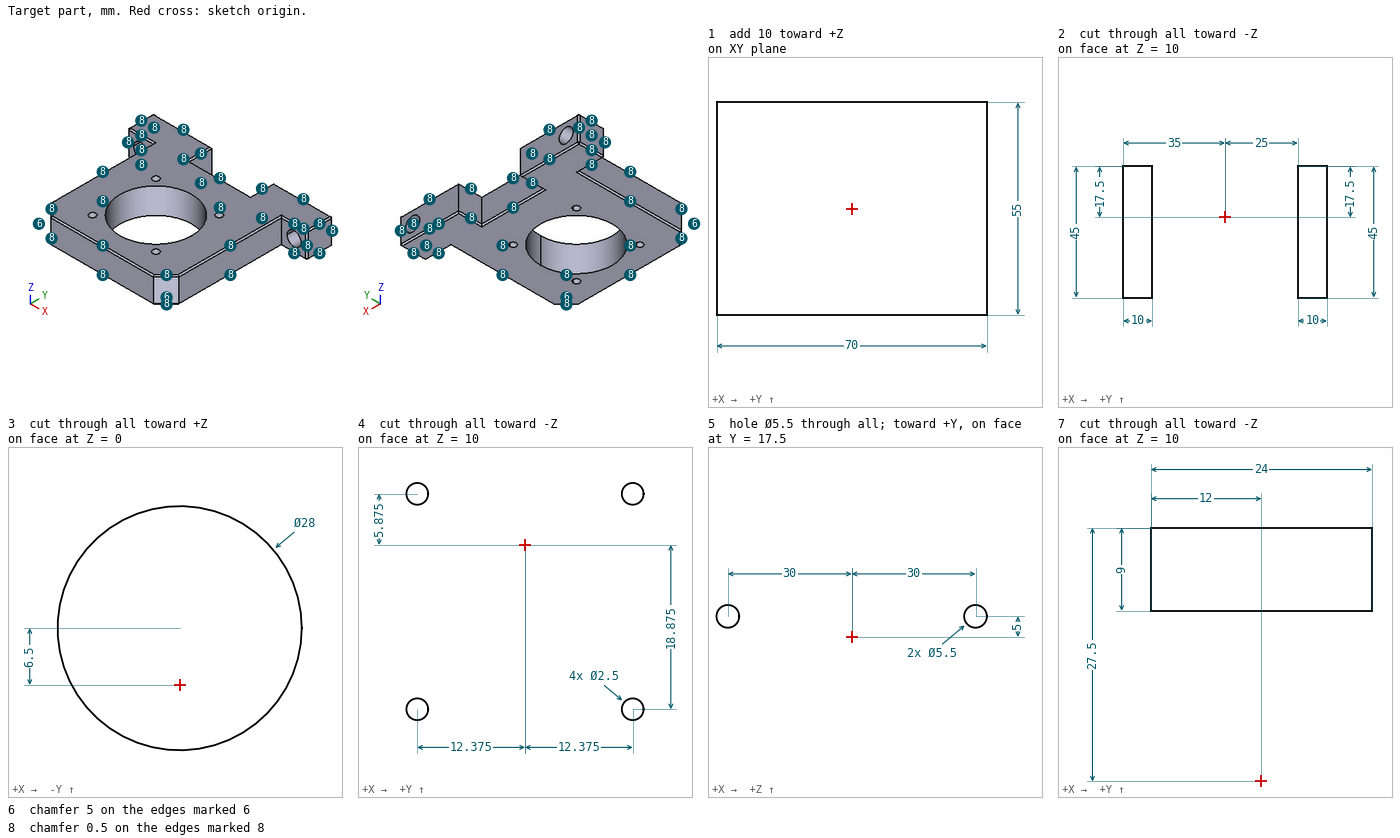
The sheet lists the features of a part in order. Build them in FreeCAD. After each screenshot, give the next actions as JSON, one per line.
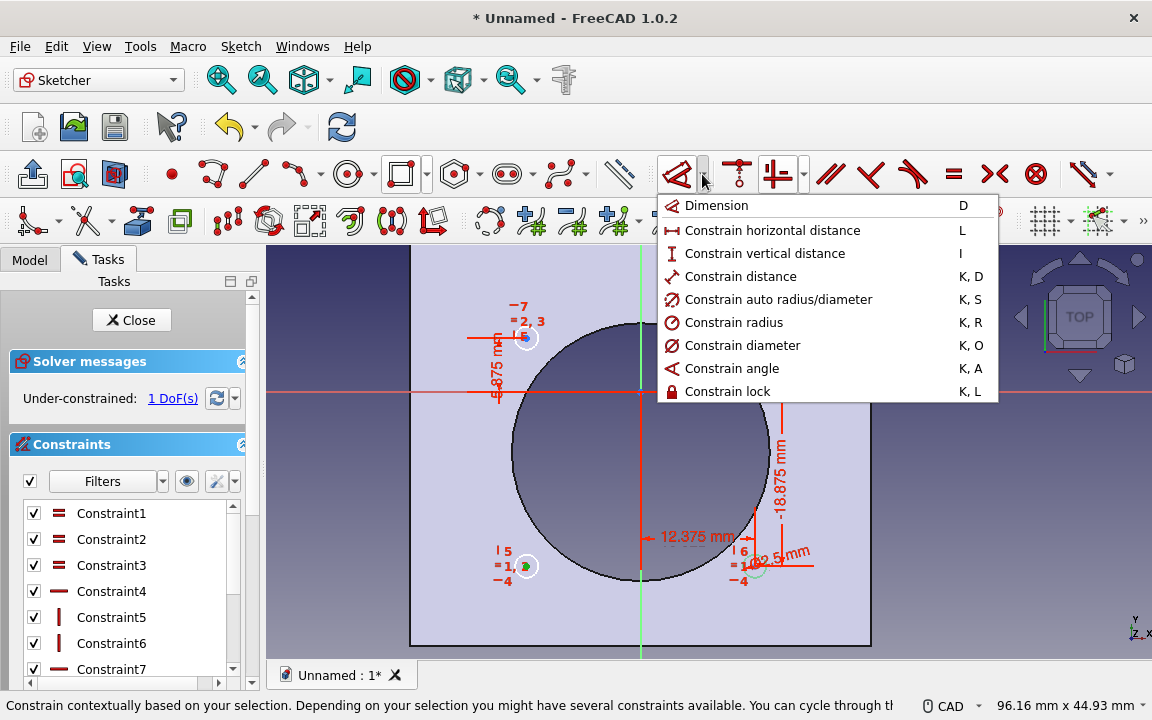
{"action": "left_click", "coordinate": [828, 230]}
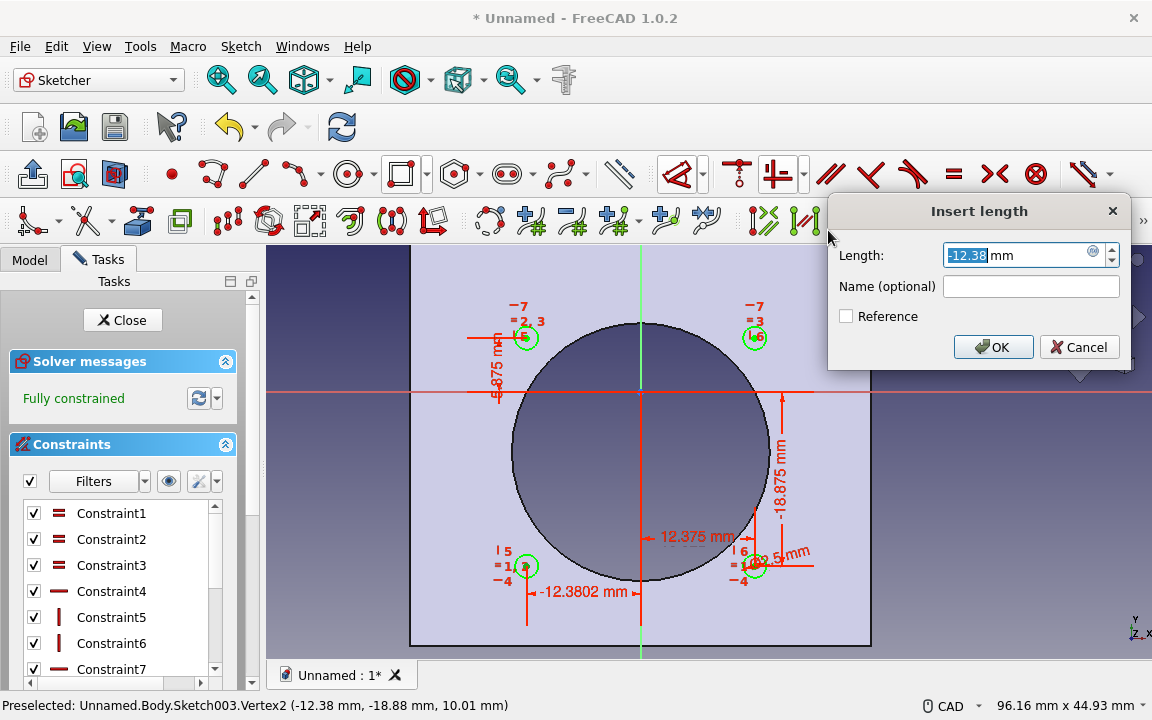
{"action": "type", "text": "-12.375"}
{"action": "key", "text": "Return"}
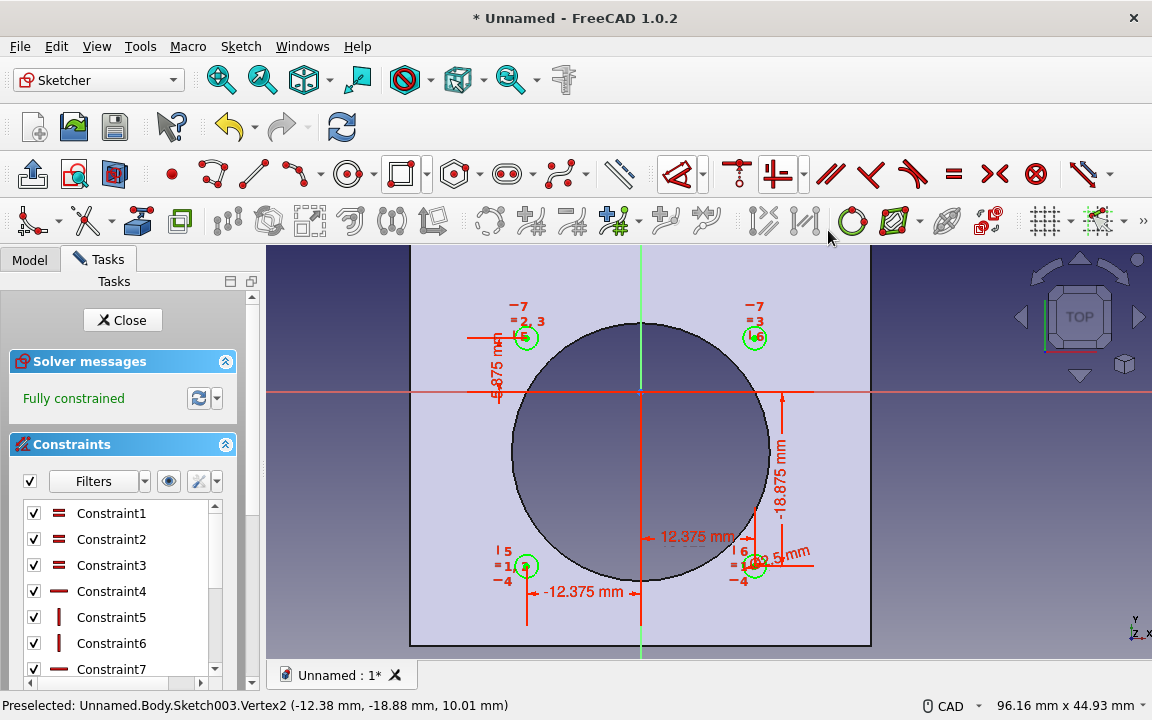
{"action": "left_click", "coordinate": [123, 320]}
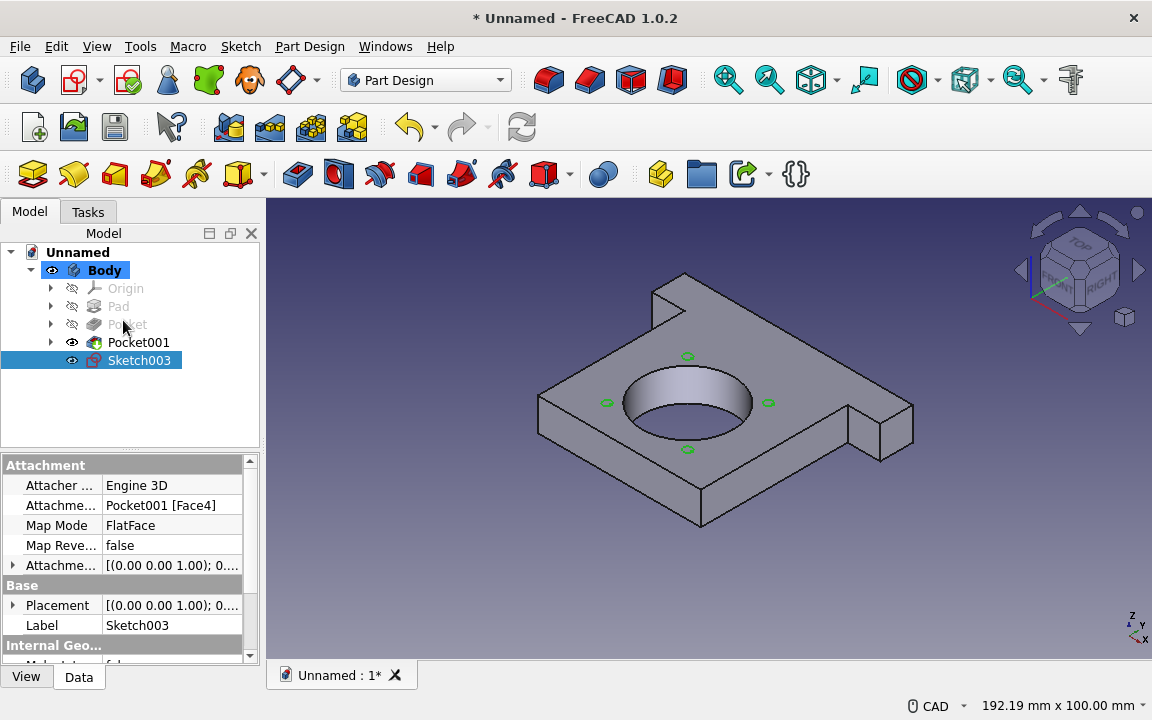
{"action": "left_click", "coordinate": [298, 174]}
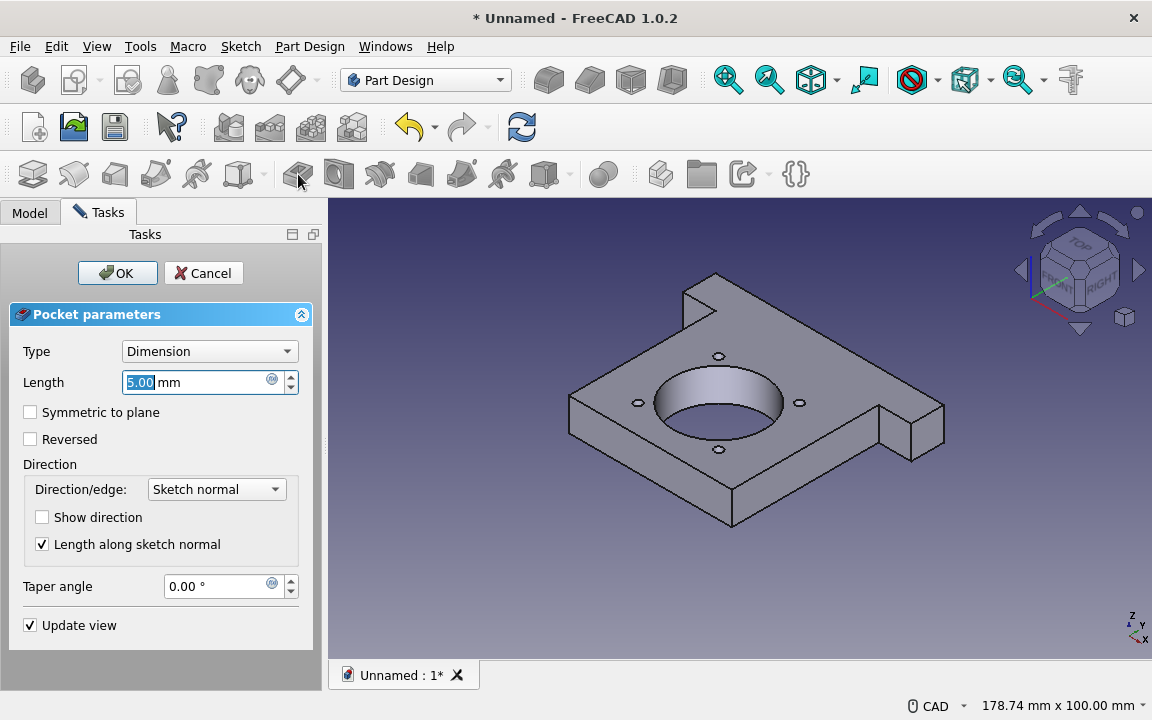
{"action": "left_click", "coordinate": [210, 352]}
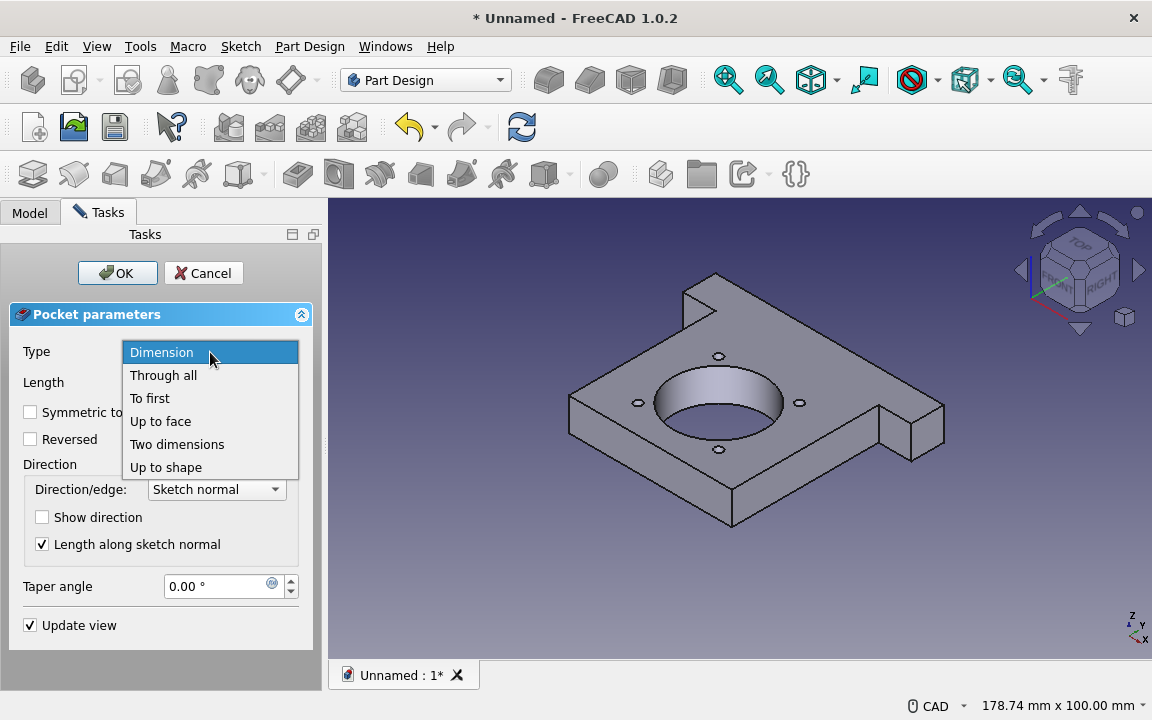
{"action": "left_click", "coordinate": [208, 376]}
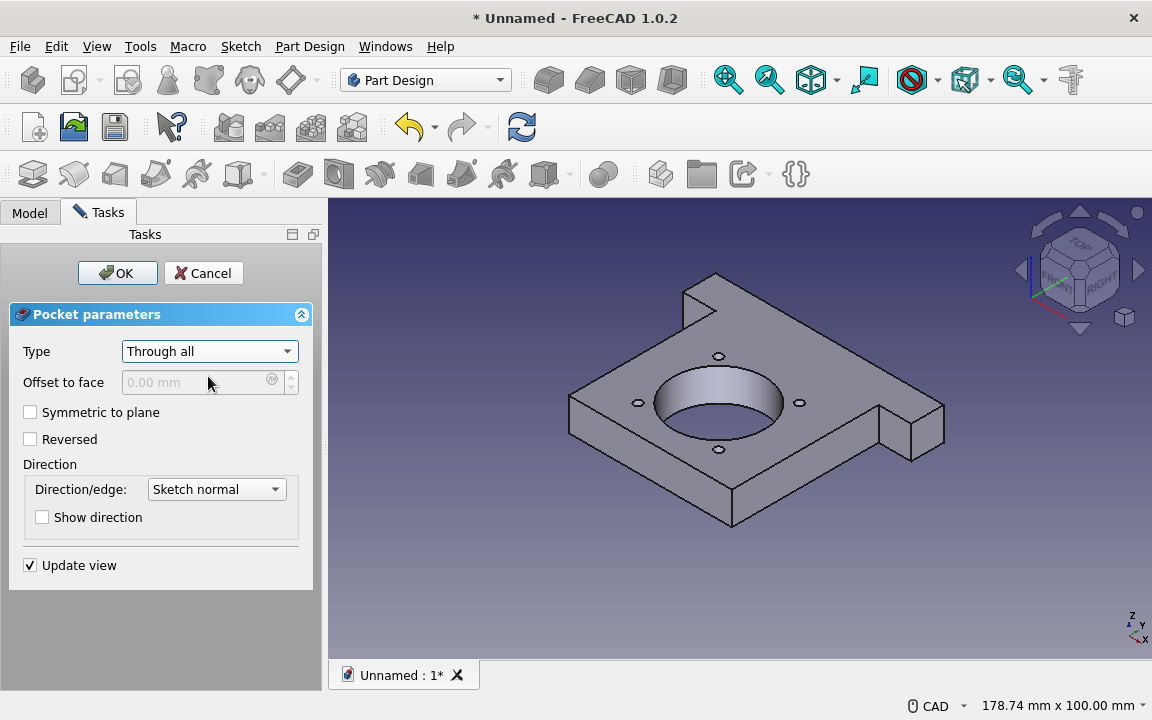
{"action": "left_click", "coordinate": [118, 273]}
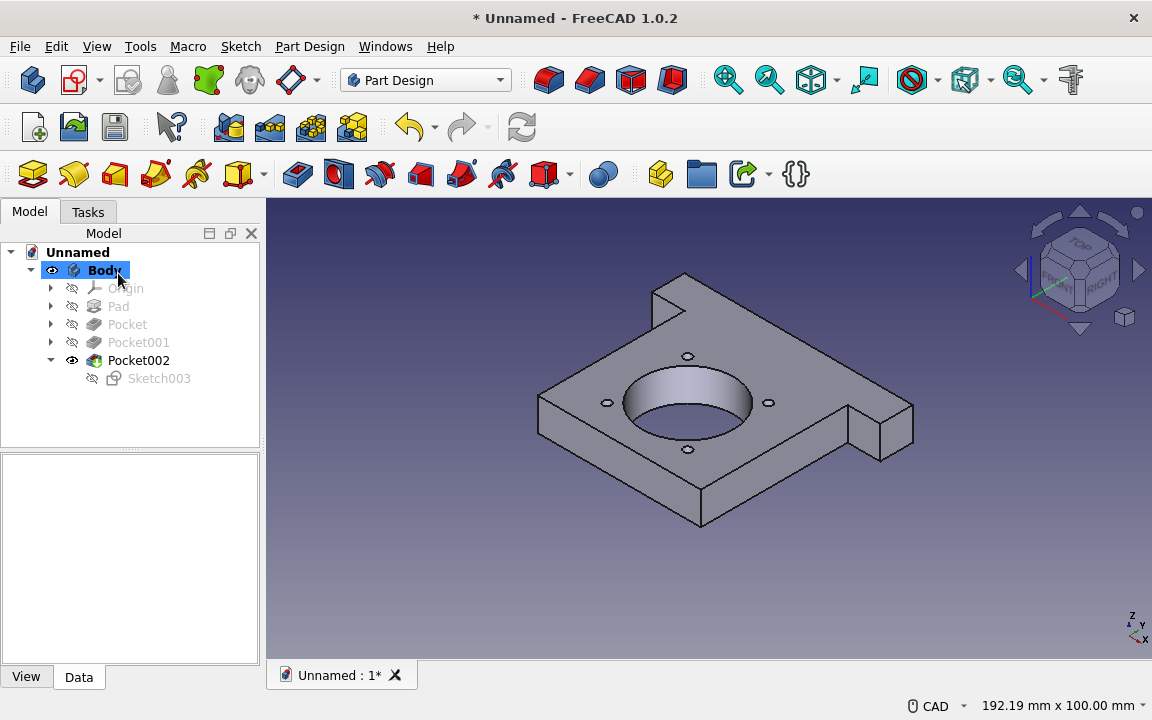
{"action": "left_click", "coordinate": [864, 432]}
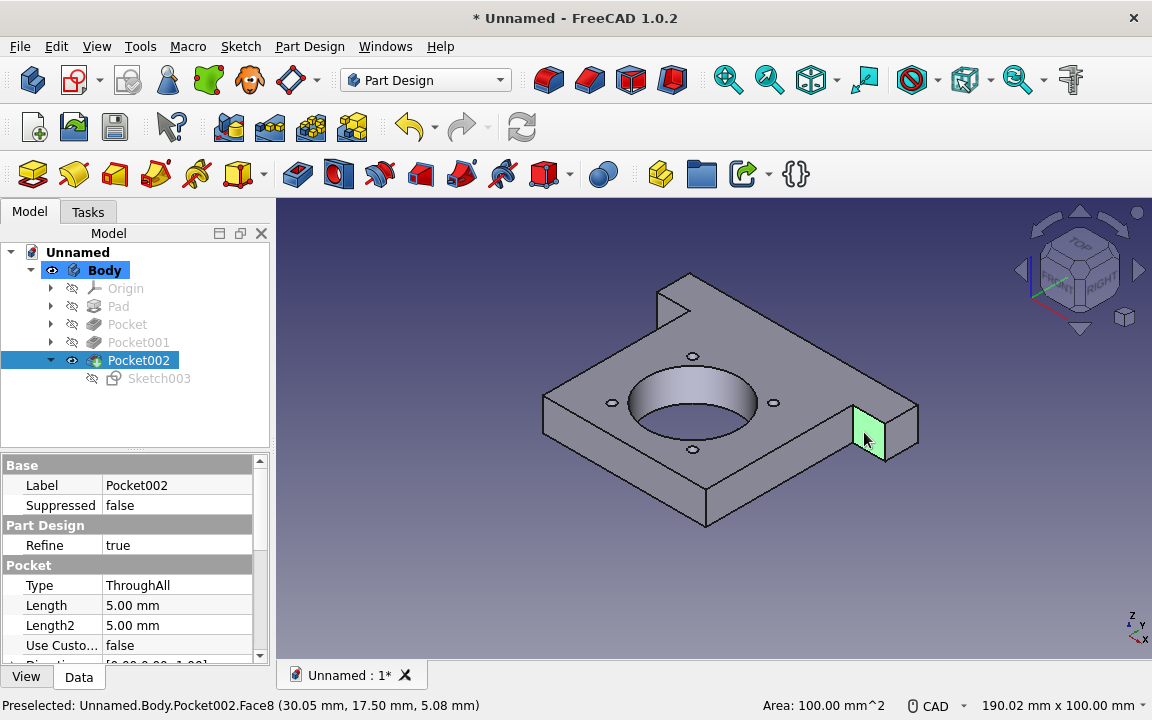
{"action": "left_click", "coordinate": [74, 80]}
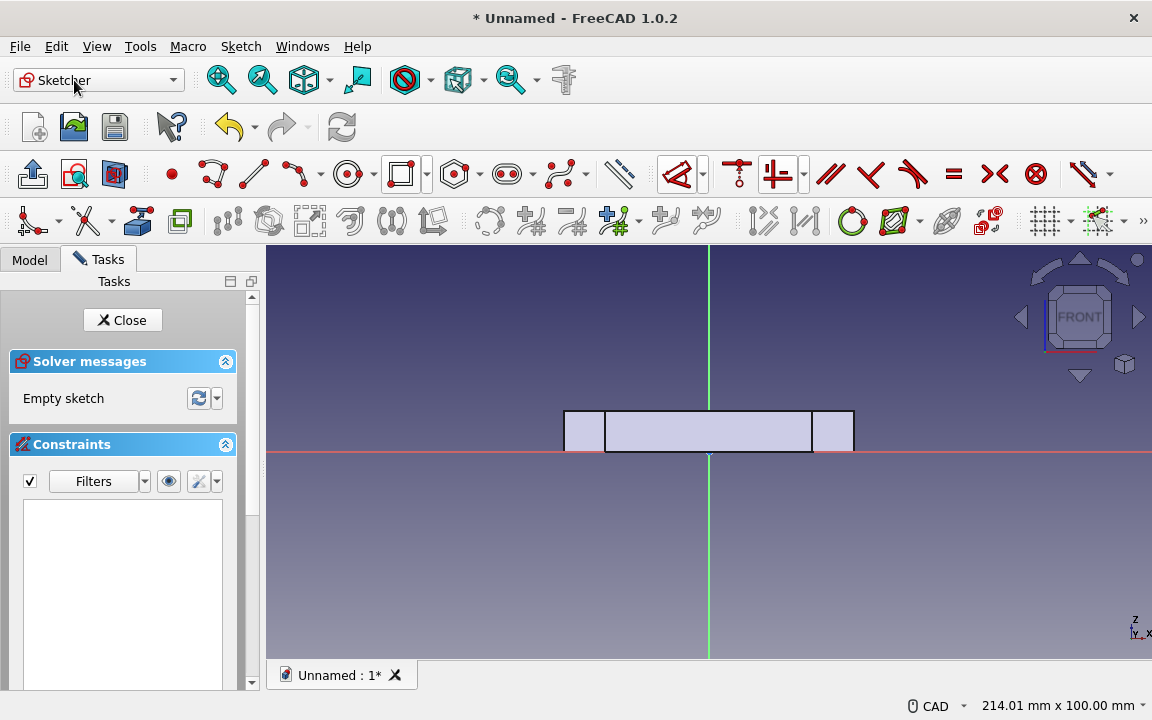
{"action": "scroll", "coordinate": [792, 416], "scroll_direction": "up", "scroll_amount": 3}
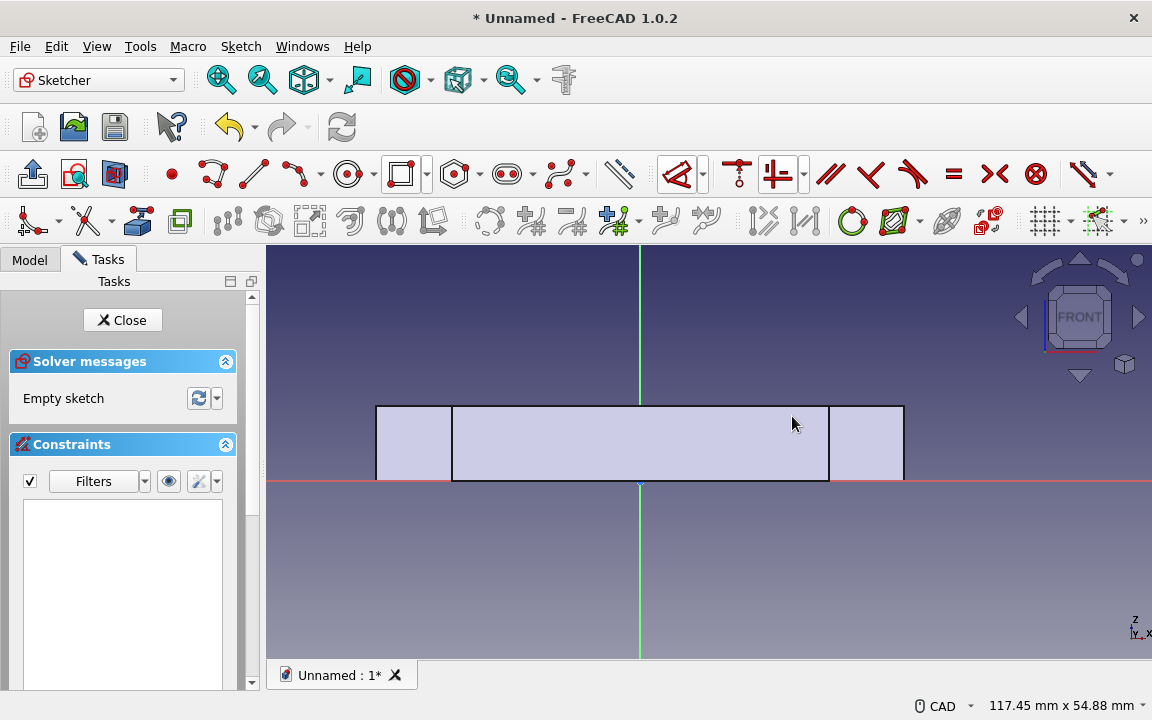
{"action": "left_click", "coordinate": [348, 174]}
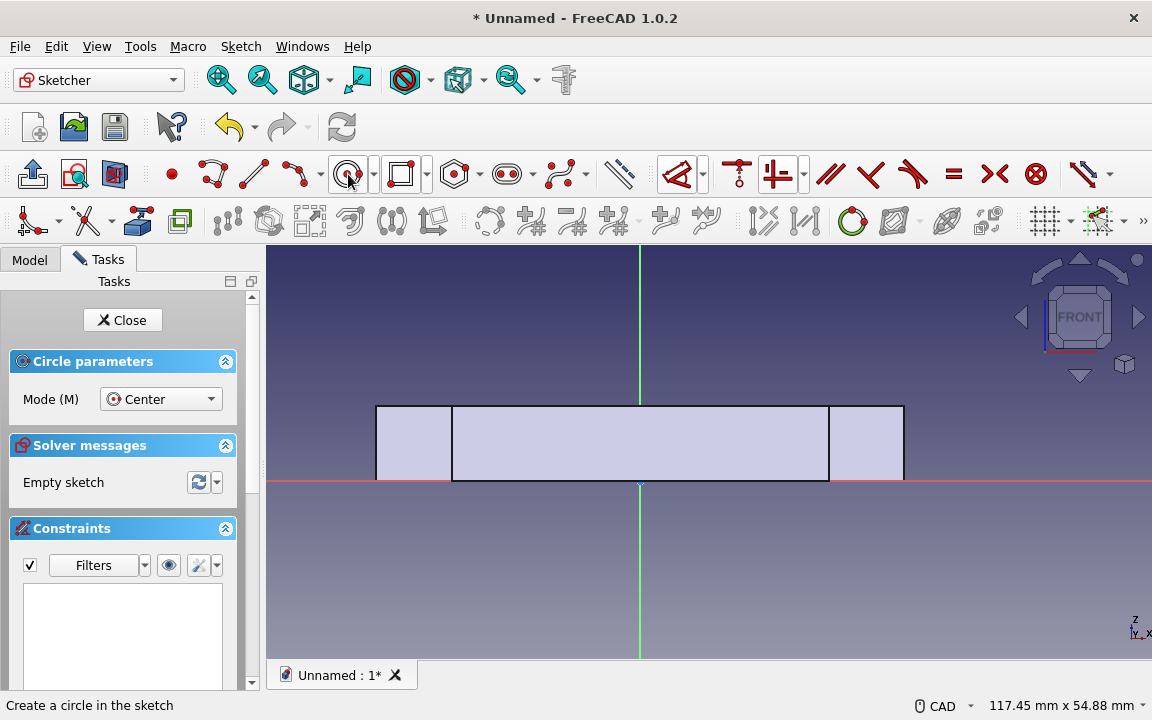
{"action": "left_click", "coordinate": [867, 444]}
{"action": "left_click", "coordinate": [881, 429]}